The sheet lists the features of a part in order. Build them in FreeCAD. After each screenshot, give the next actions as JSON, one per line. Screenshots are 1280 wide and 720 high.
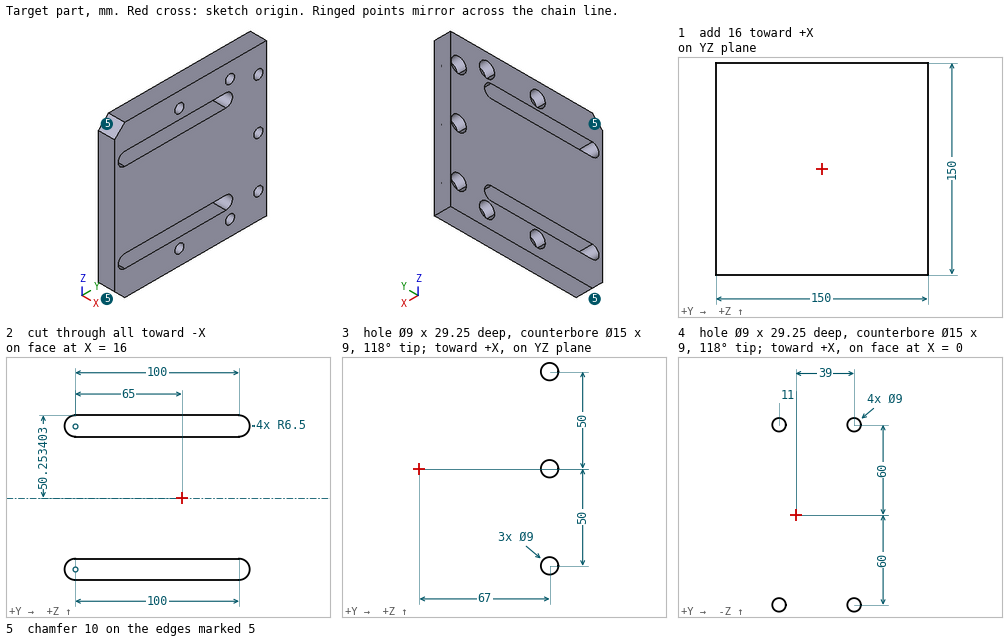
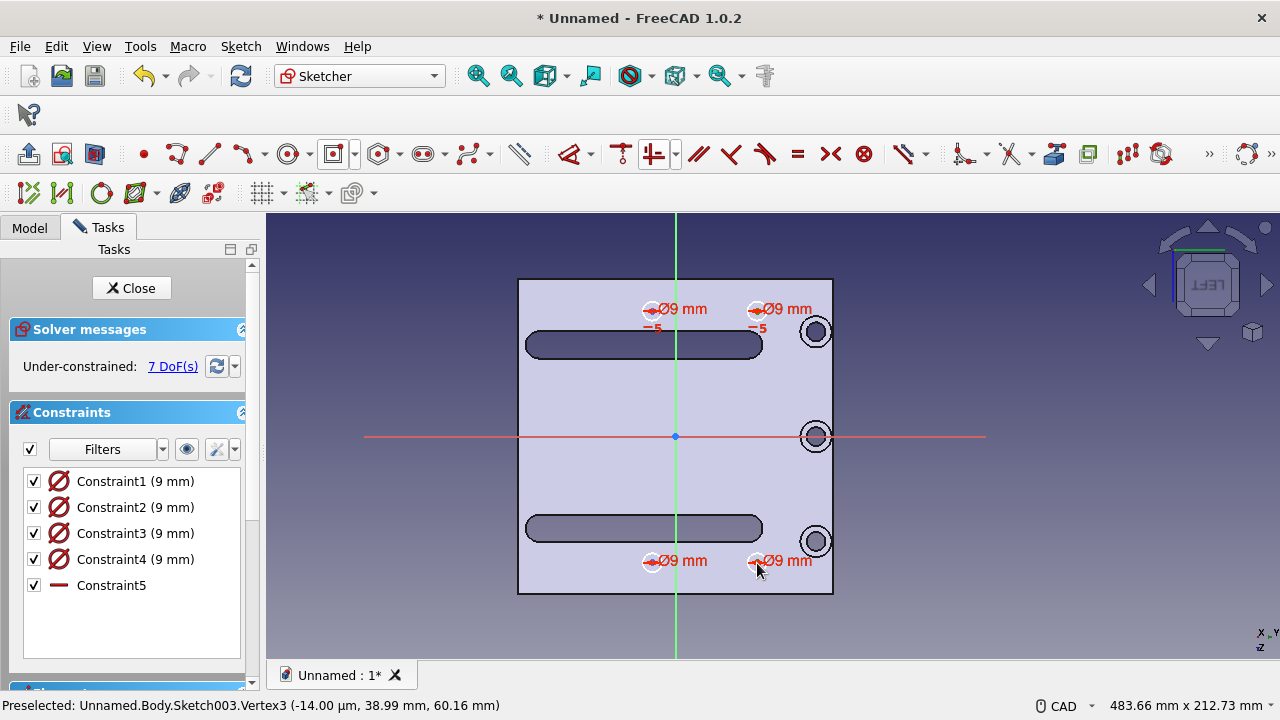
{"action": "left_click", "coordinate": [676, 154]}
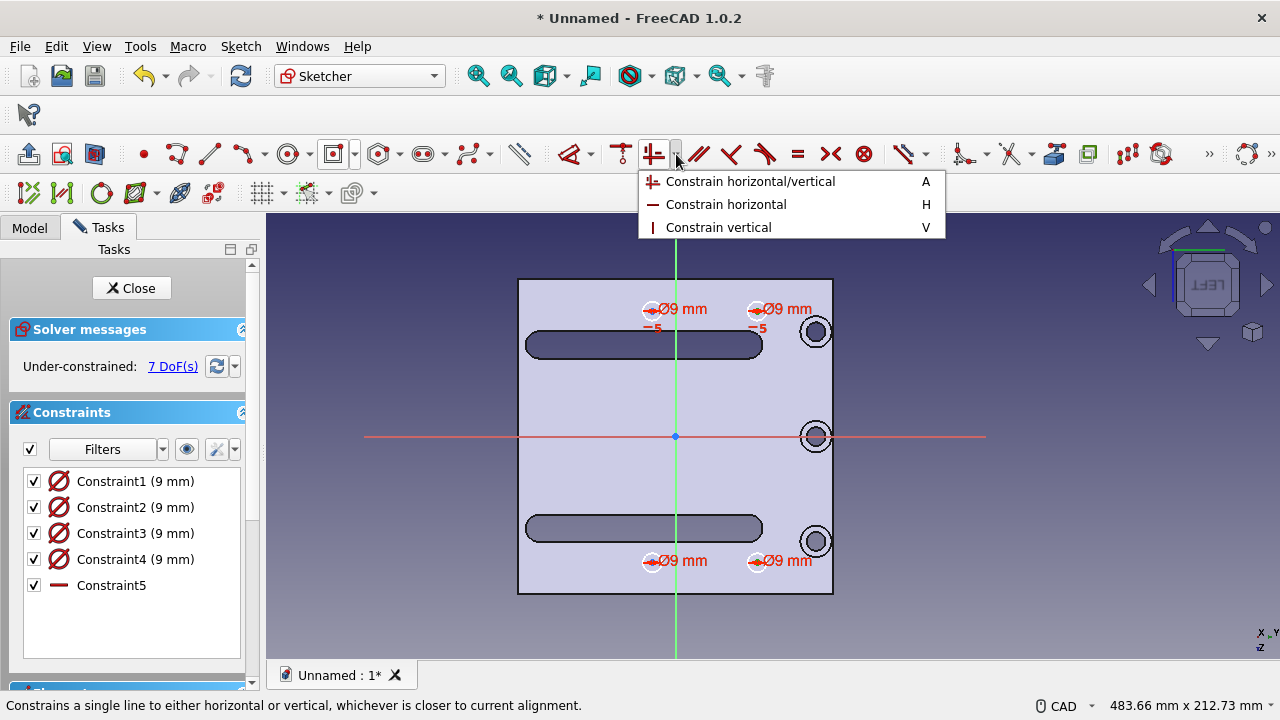
{"action": "left_click", "coordinate": [792, 228]}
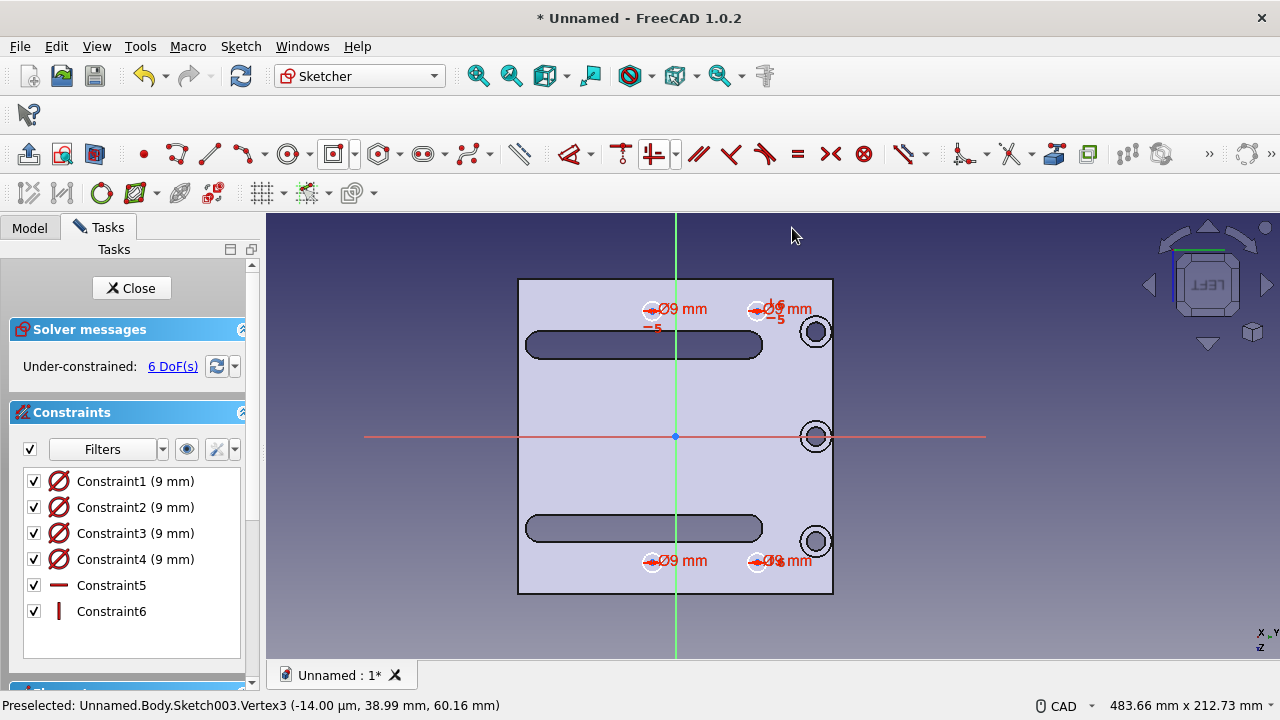
{"action": "left_click", "coordinate": [652, 311]}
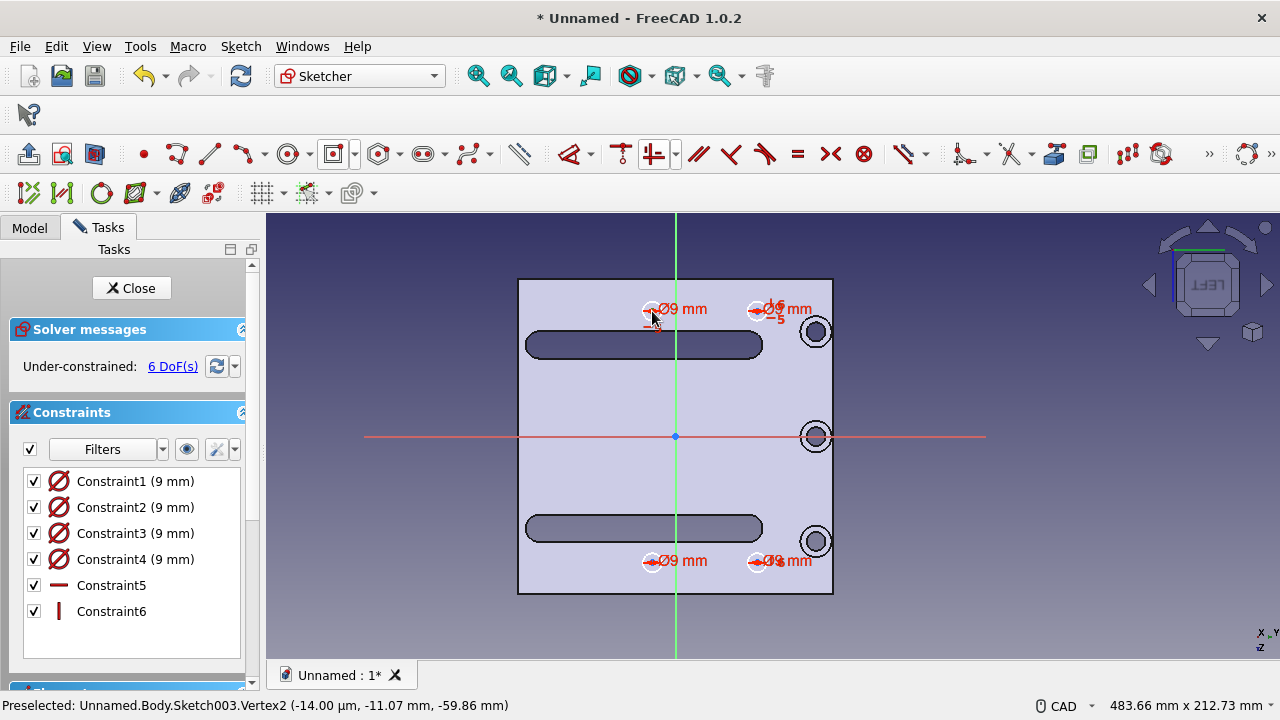
{"action": "left_click", "coordinate": [652, 563]}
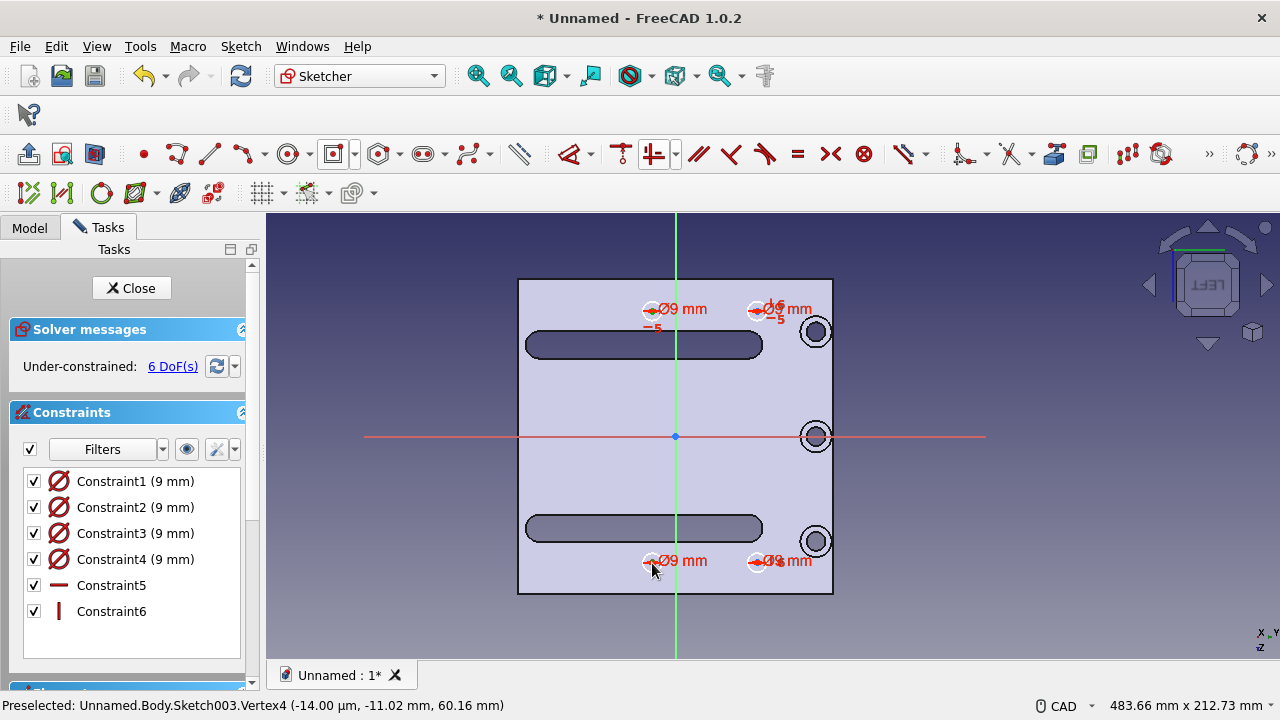
{"action": "key", "text": "v"}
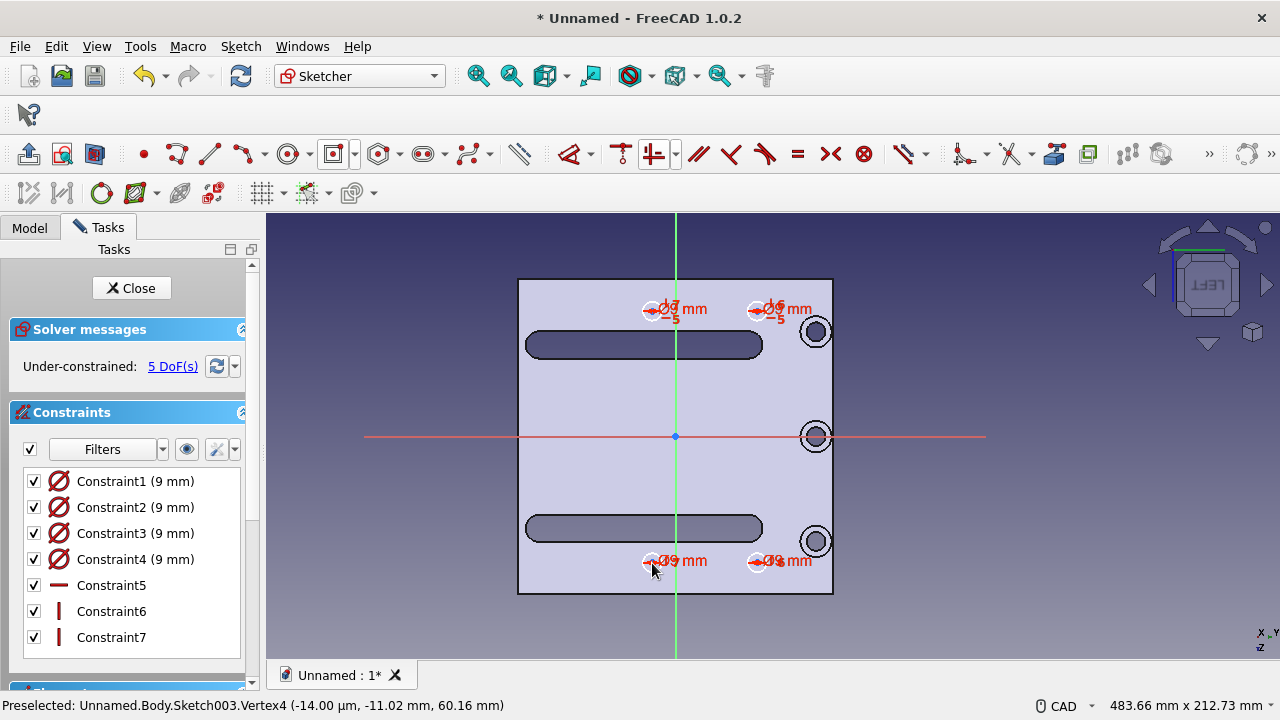
{"action": "left_click", "coordinate": [757, 563]}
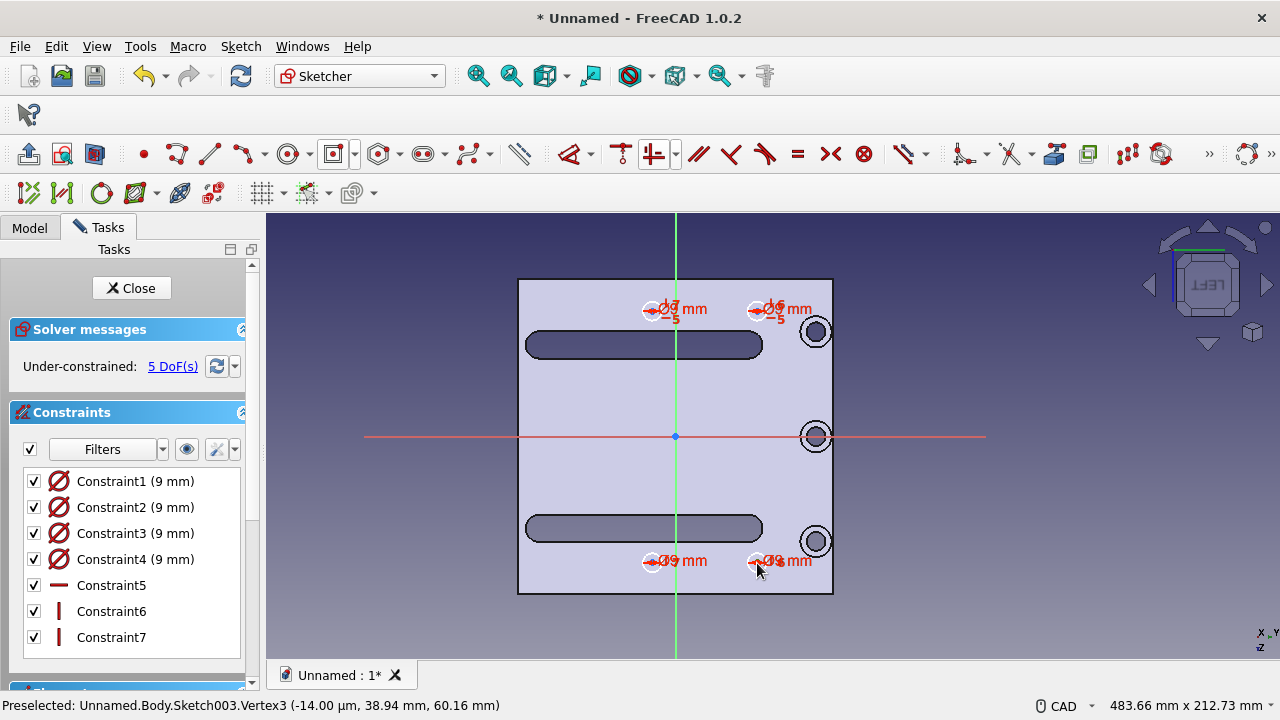
{"action": "left_click", "coordinate": [652, 563]}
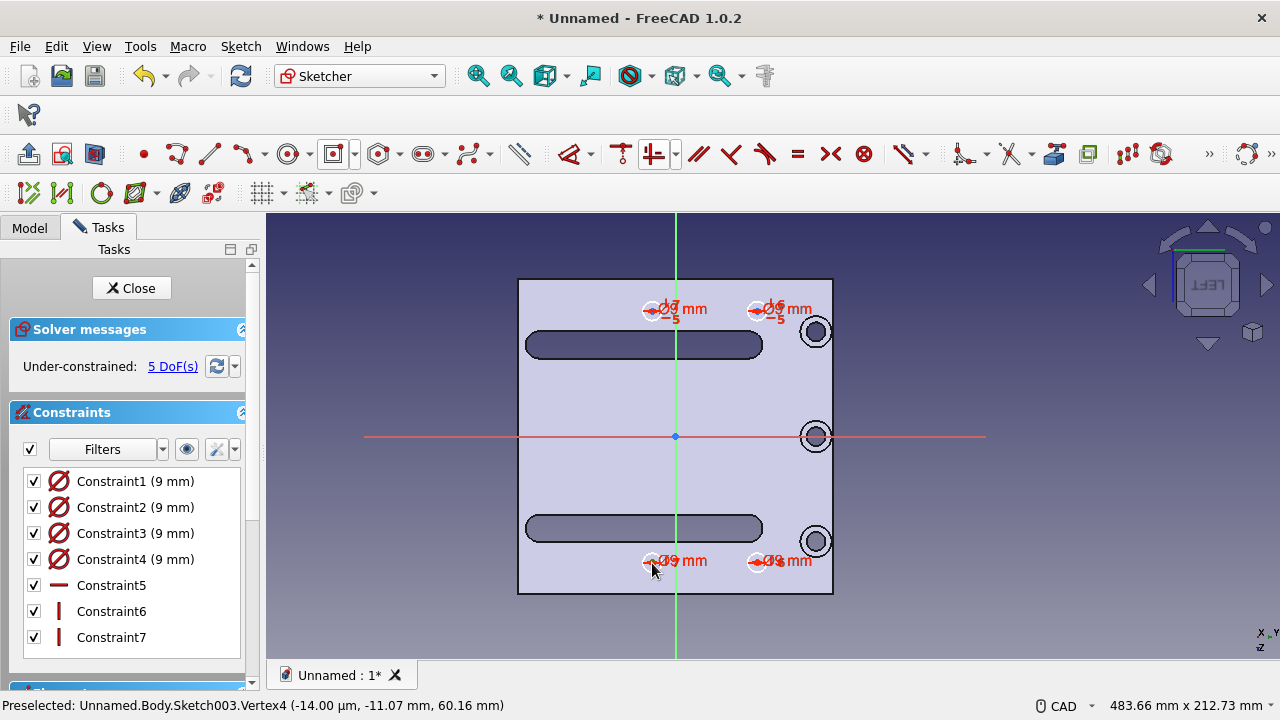
{"action": "left_click", "coordinate": [676, 154]}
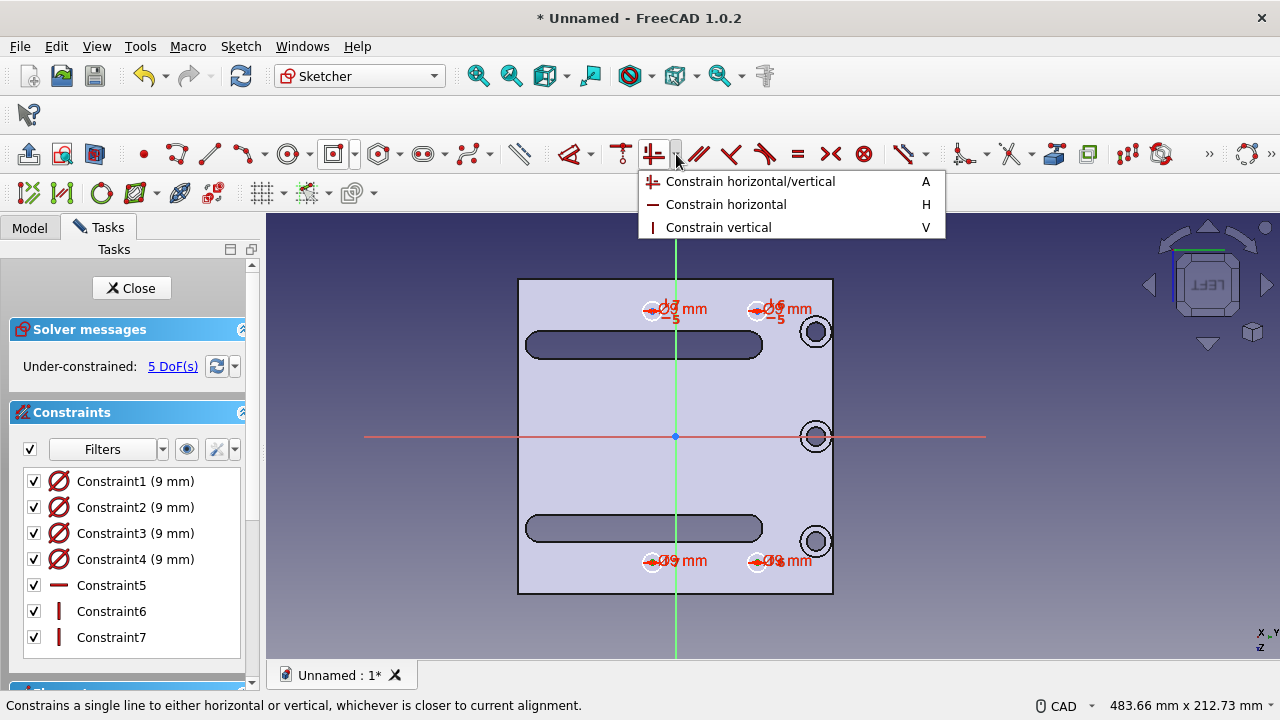
{"action": "left_click", "coordinate": [792, 204]}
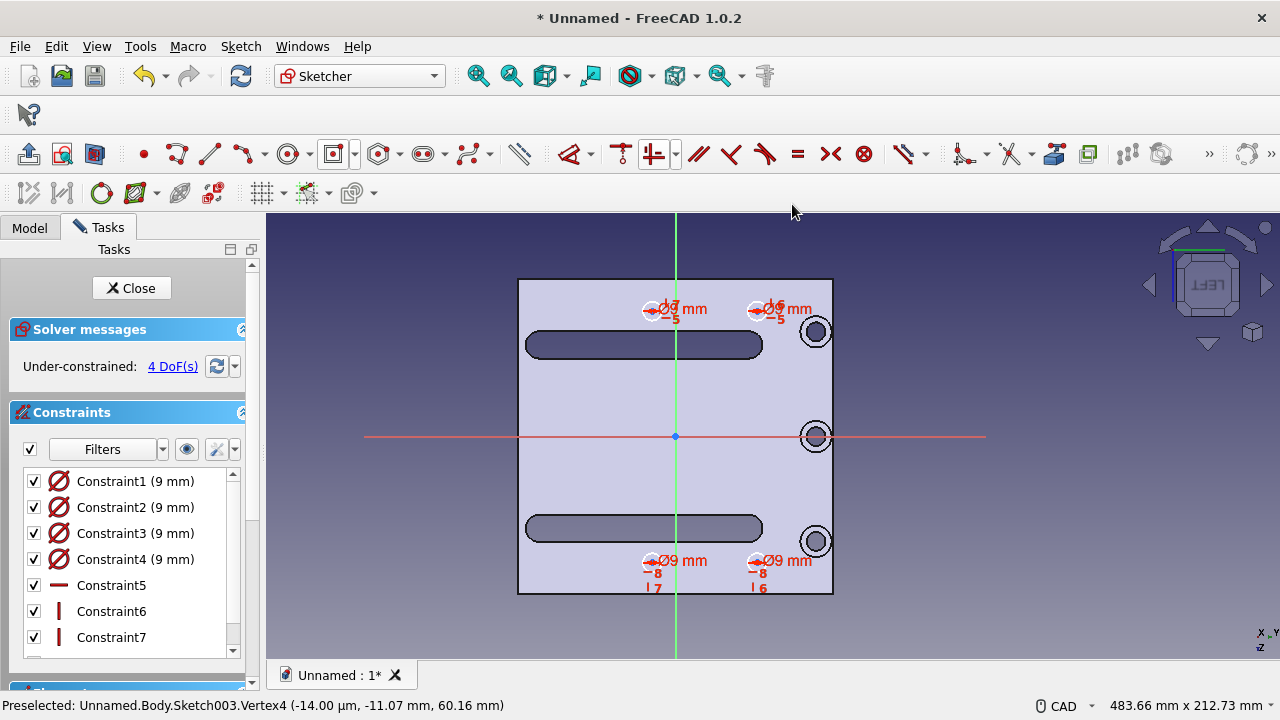
{"action": "left_click", "coordinate": [568, 154]}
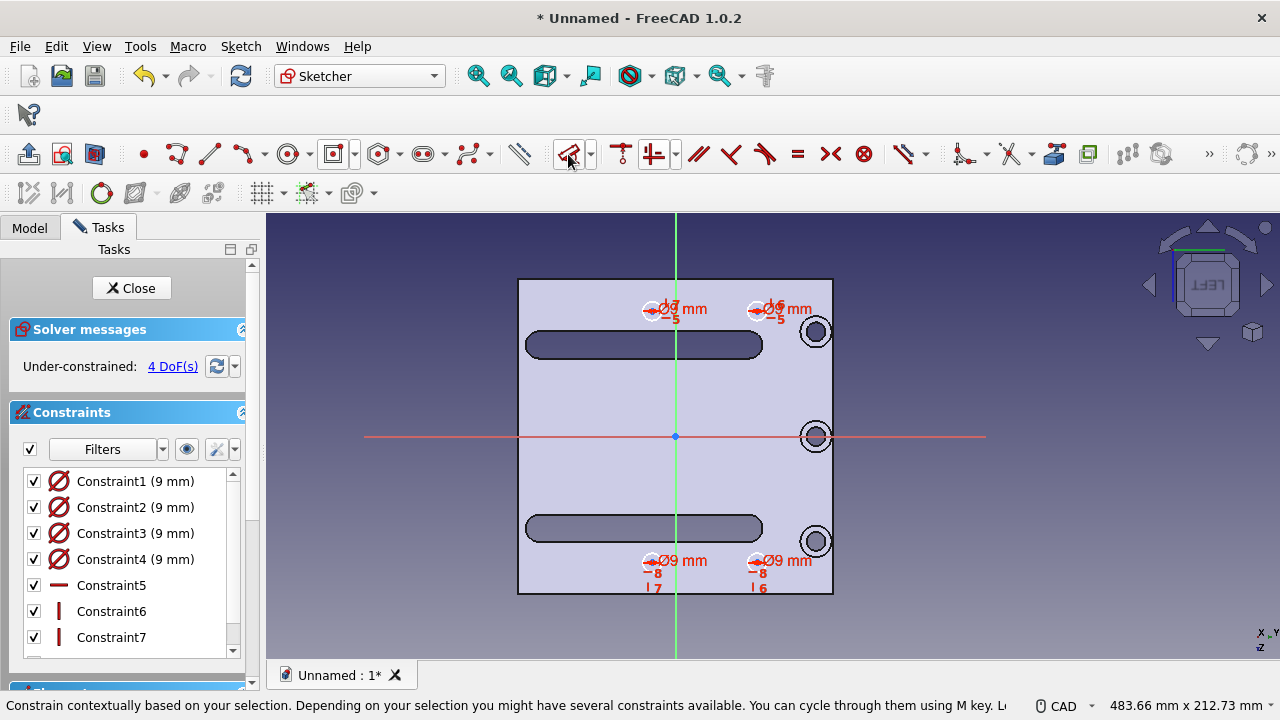
{"action": "left_click", "coordinate": [757, 311]}
{"action": "left_click", "coordinate": [716, 277]}